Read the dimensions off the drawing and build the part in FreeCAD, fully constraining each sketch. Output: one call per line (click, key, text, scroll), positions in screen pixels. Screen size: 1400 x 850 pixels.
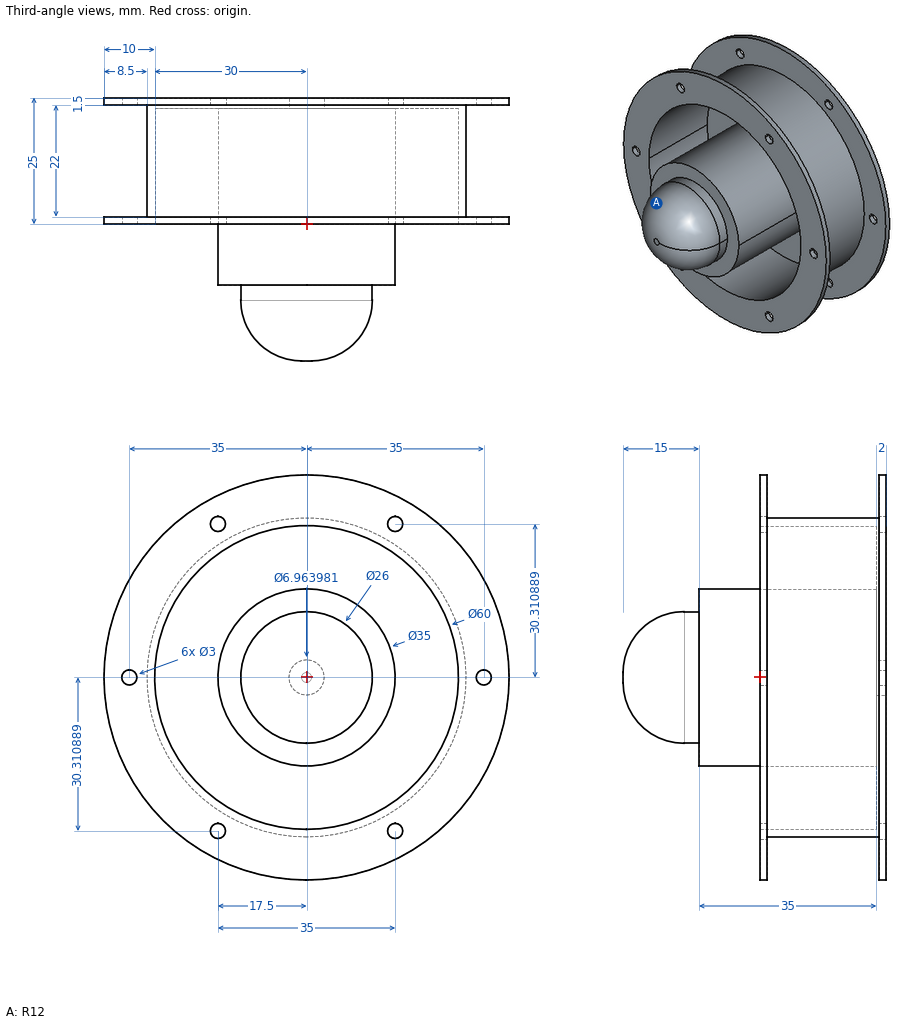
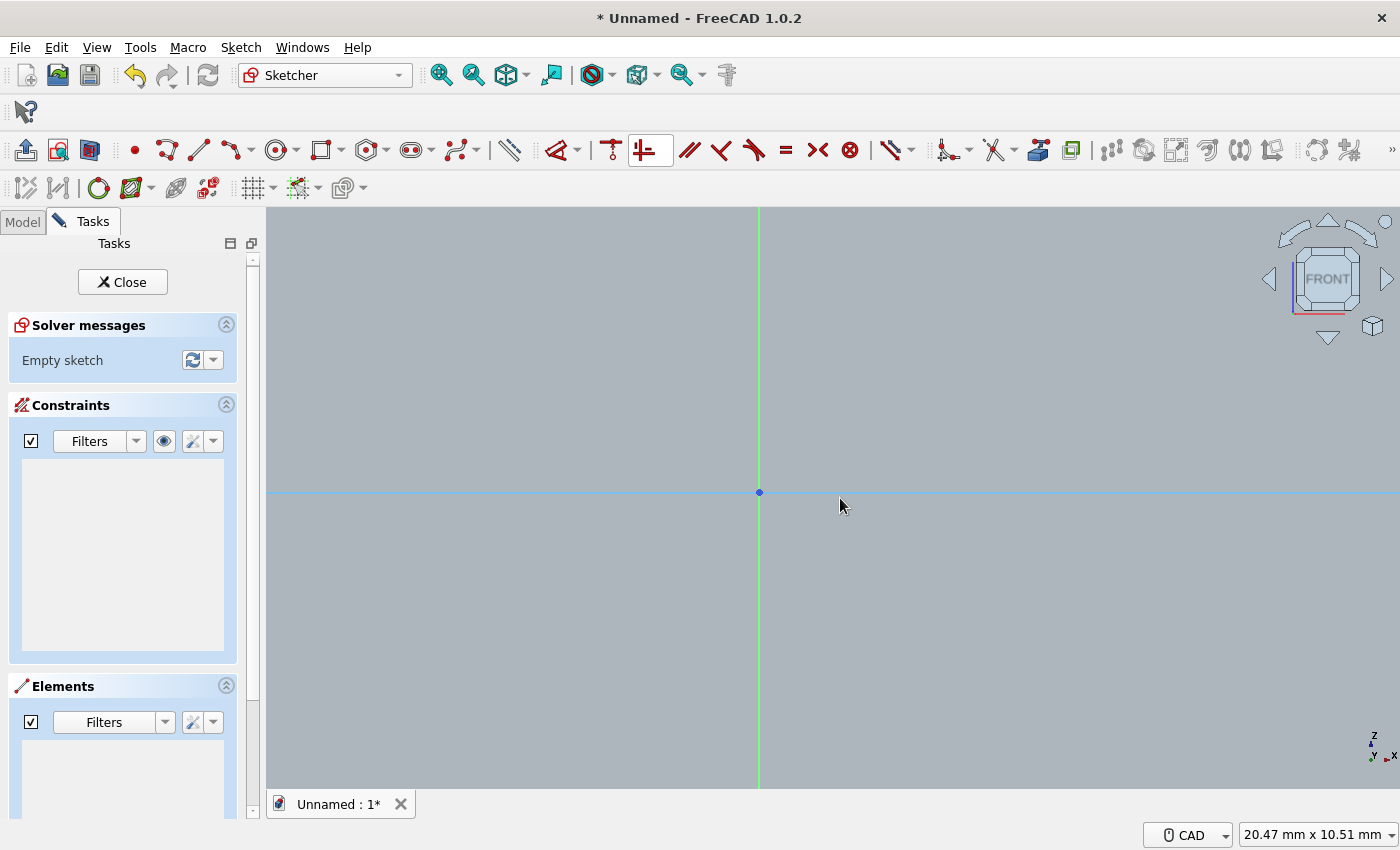
click(276, 150)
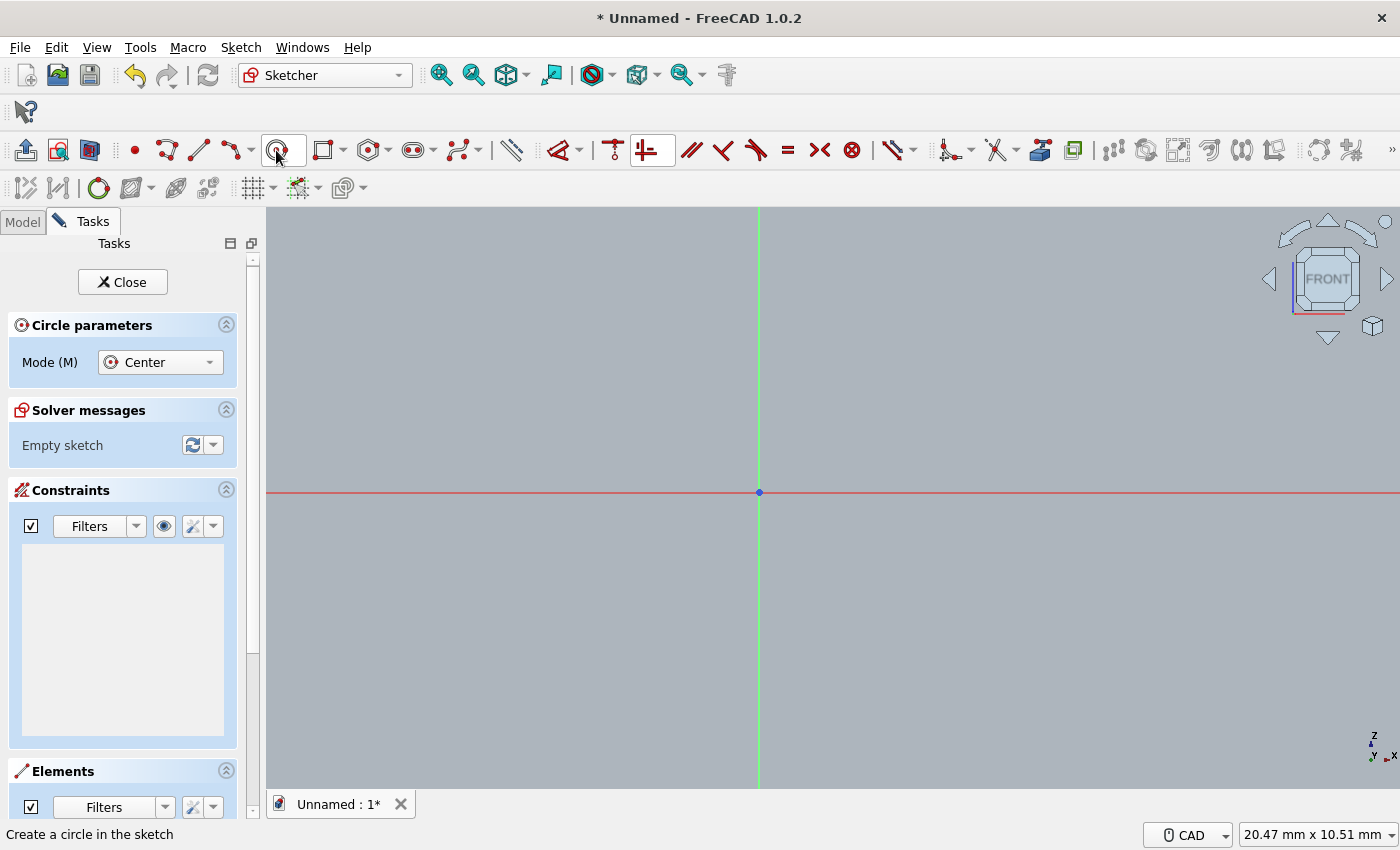
click(759, 493)
click(896, 357)
key(Escape)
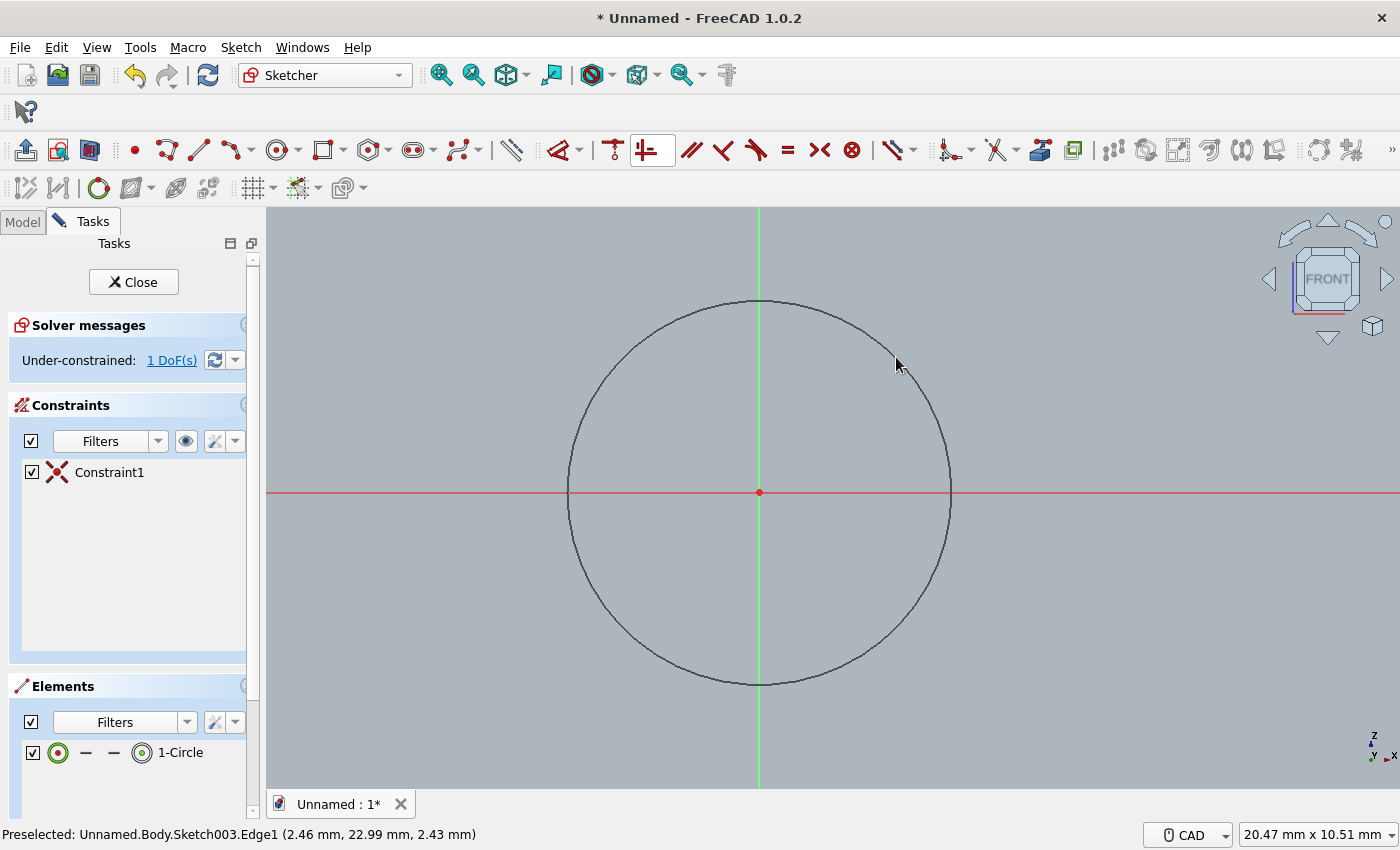
click(558, 150)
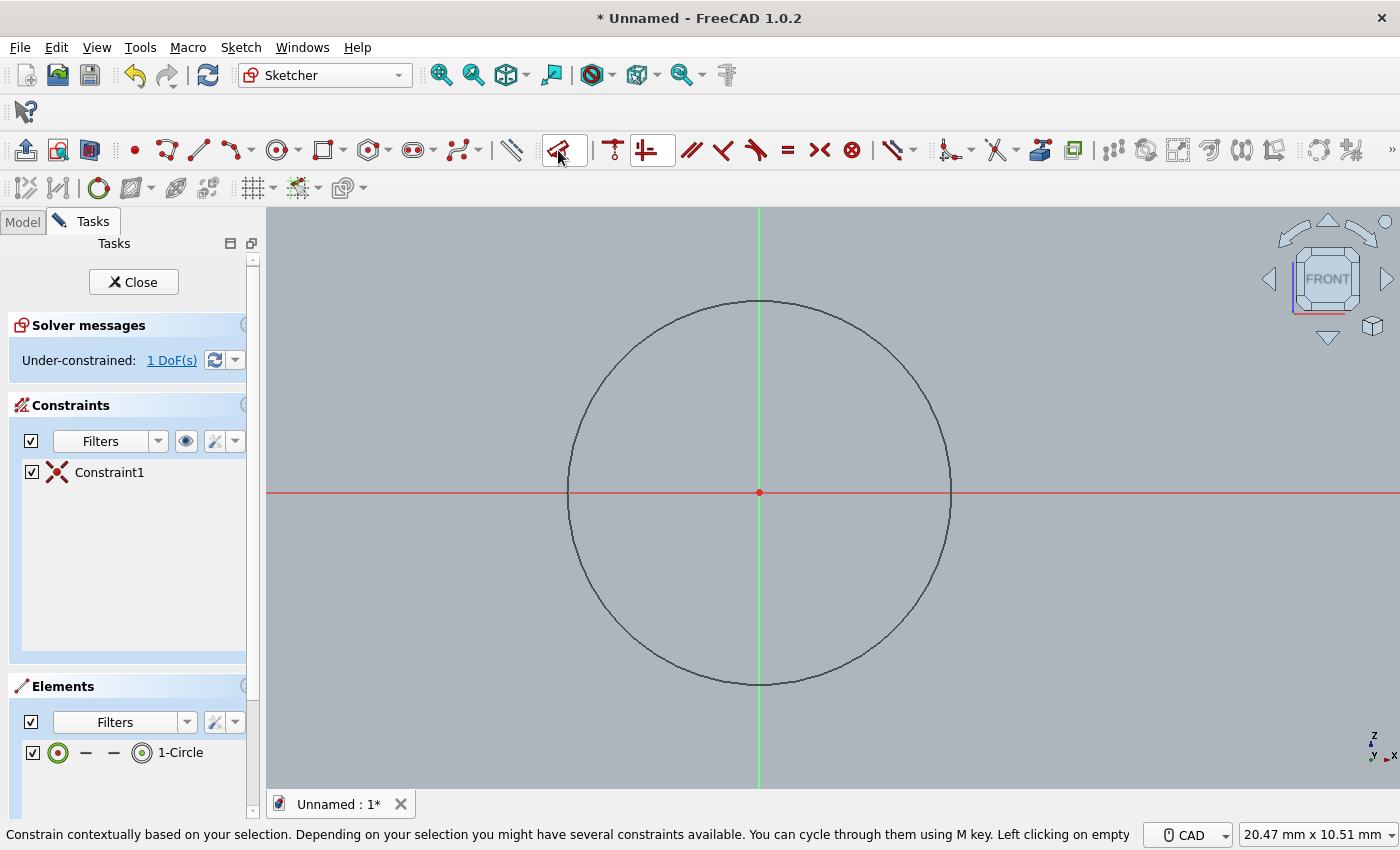
click(895, 357)
click(918, 334)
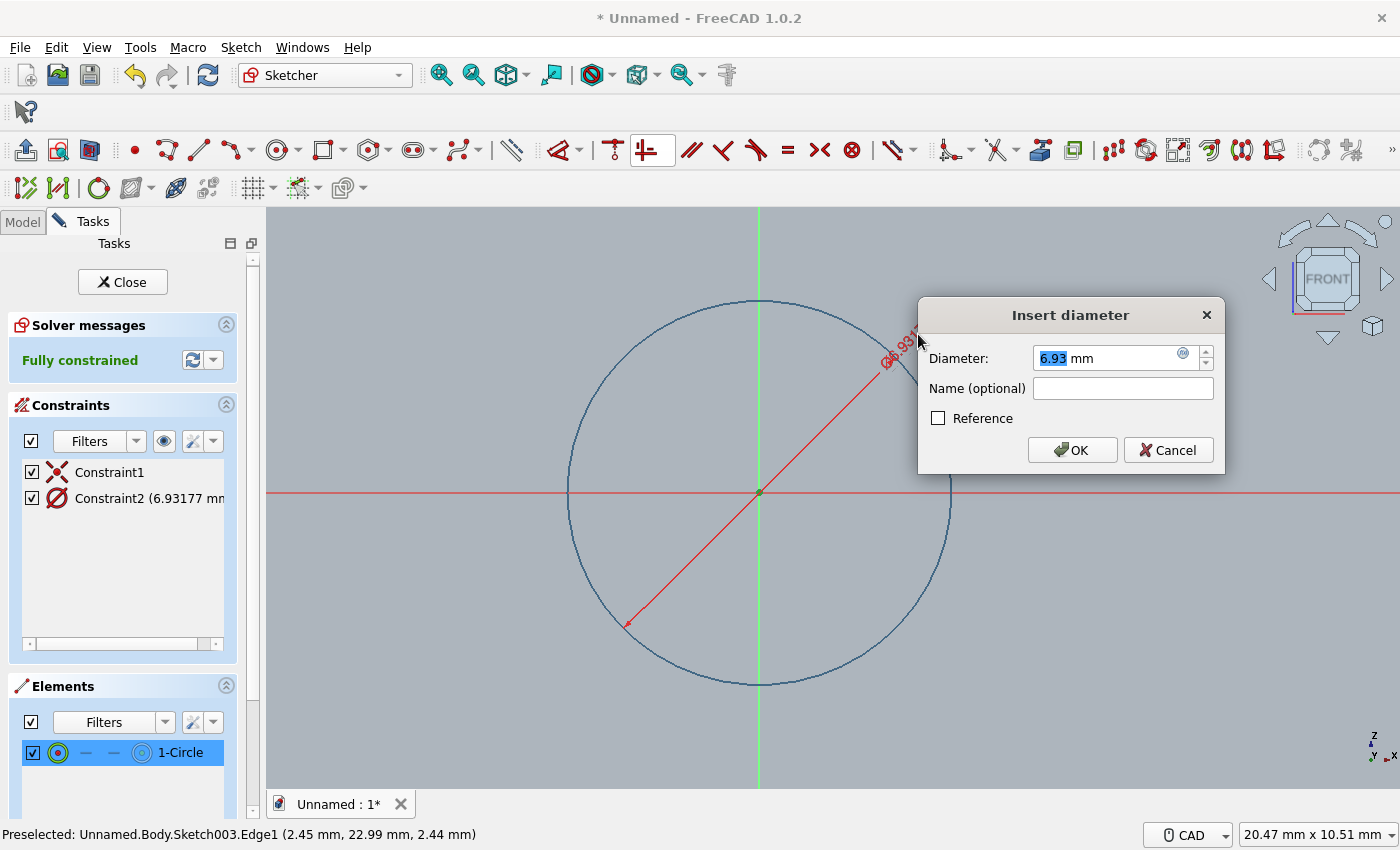
text(6.963981)
key(Return)
key(Escape)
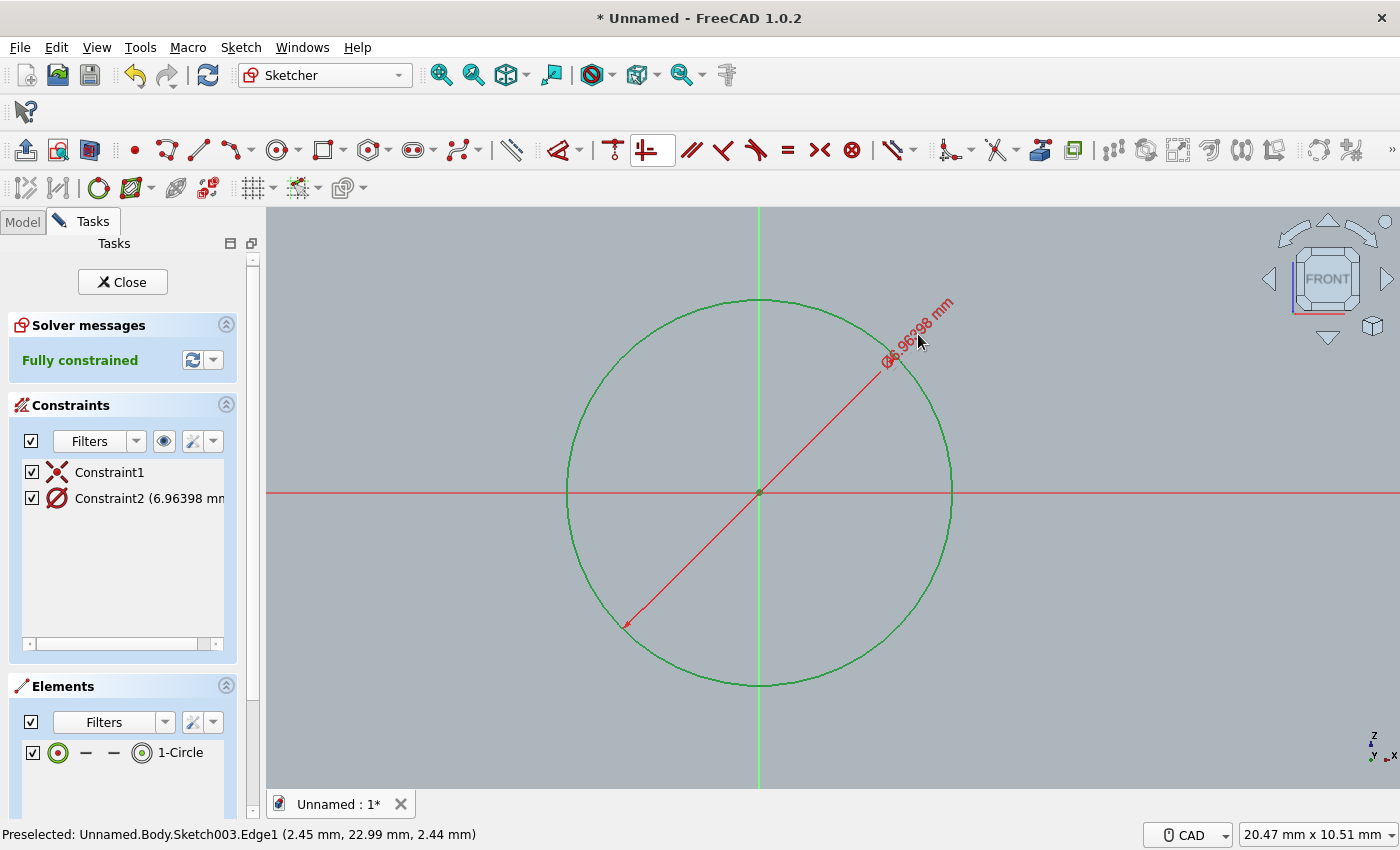
click(123, 282)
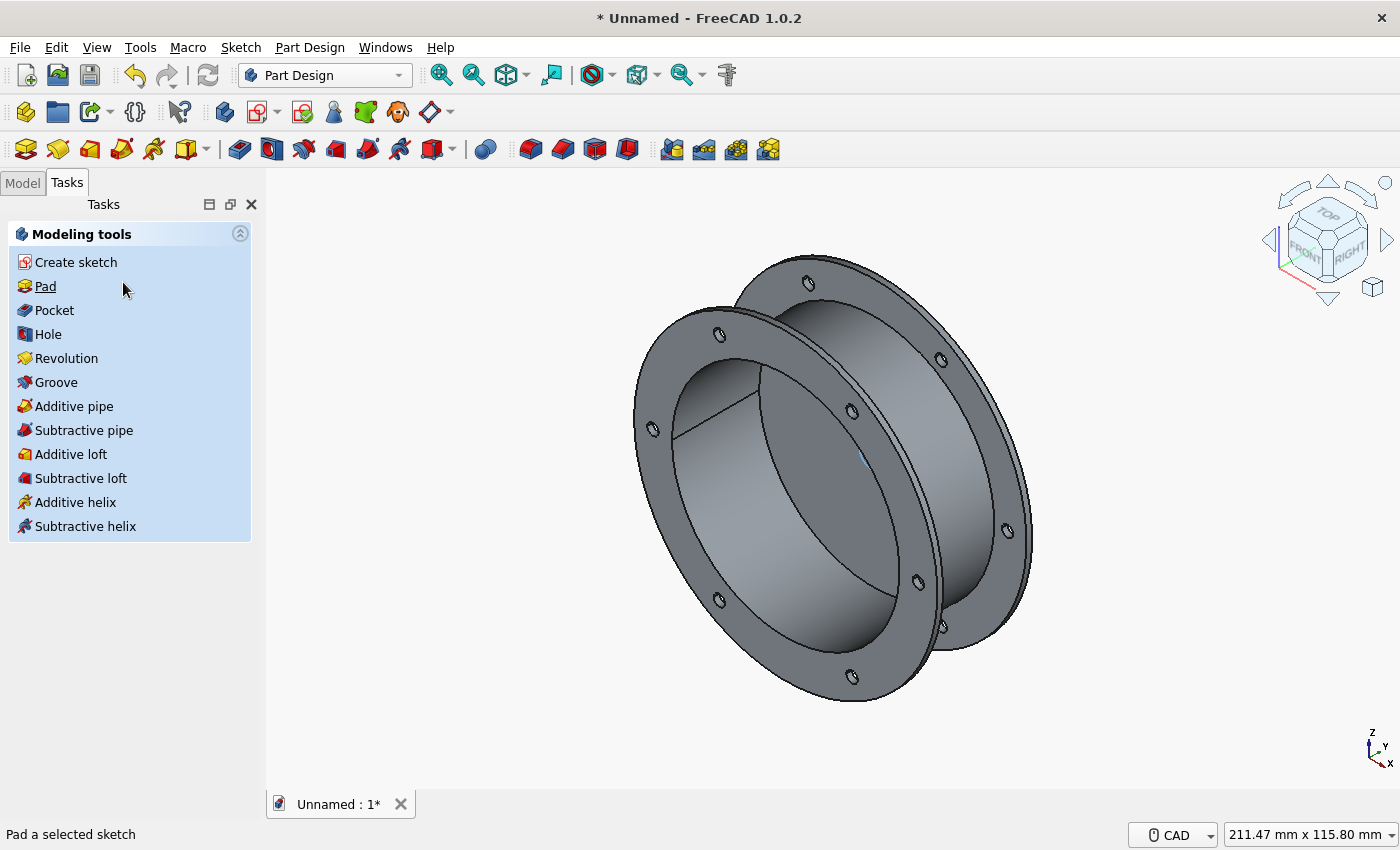
click(240, 150)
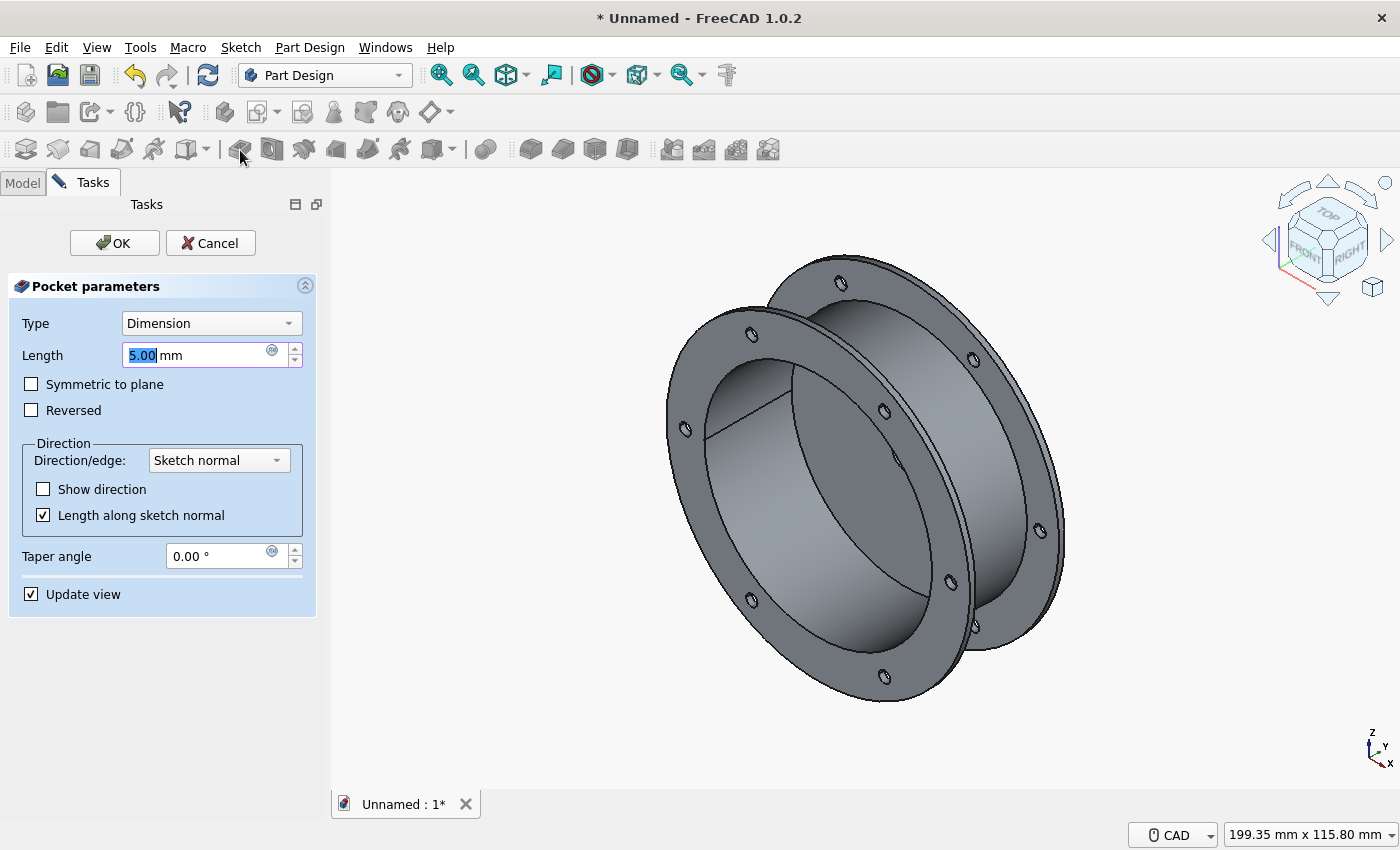
text(2)
key(Tab)